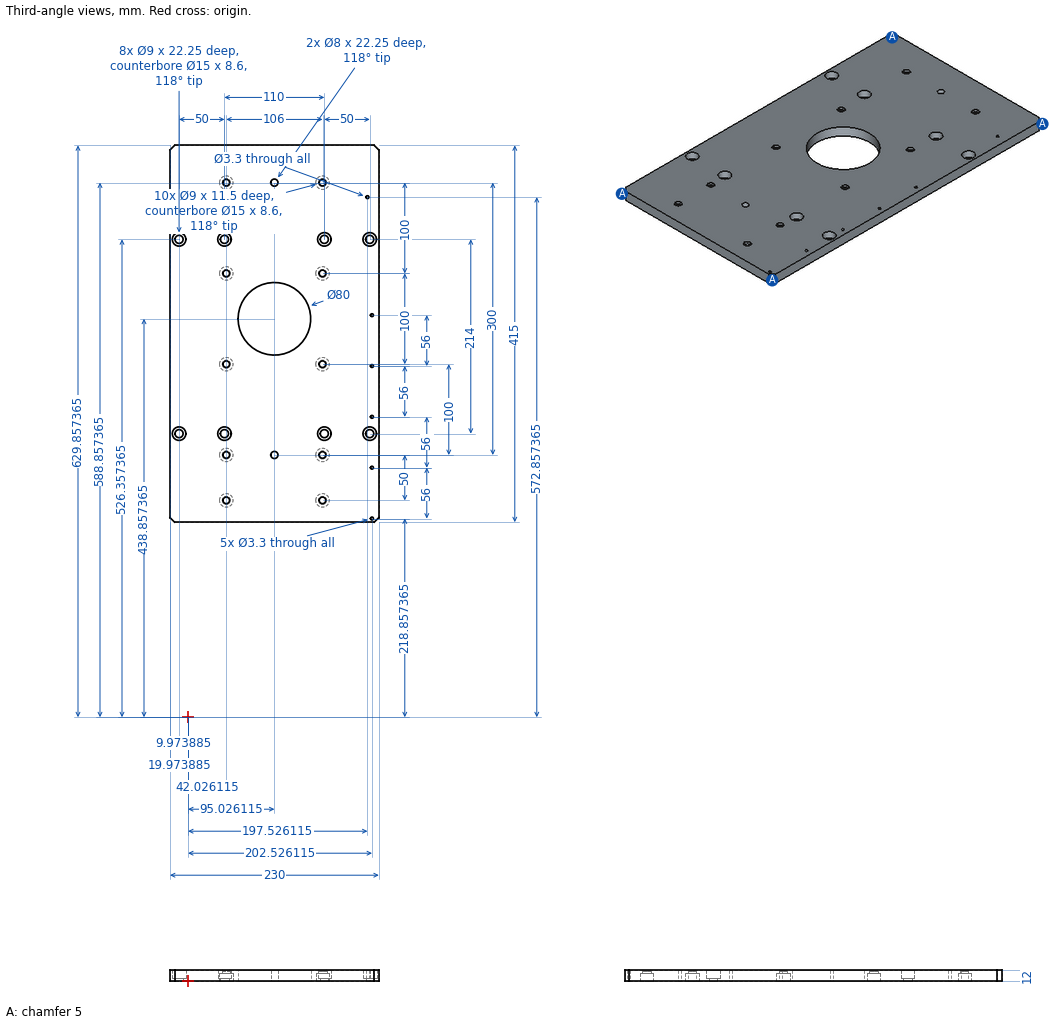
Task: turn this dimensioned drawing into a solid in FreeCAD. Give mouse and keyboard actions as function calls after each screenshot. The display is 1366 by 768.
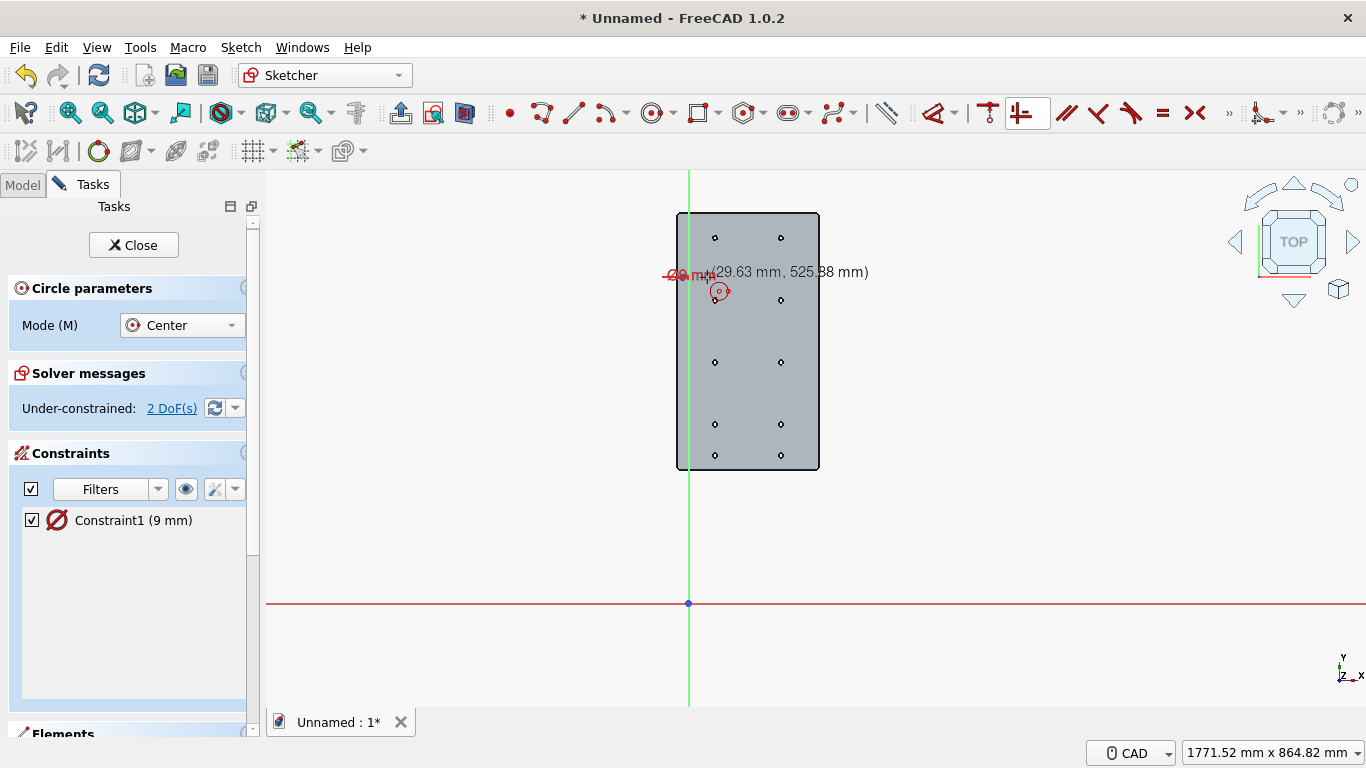
click(714, 277)
move(716, 275)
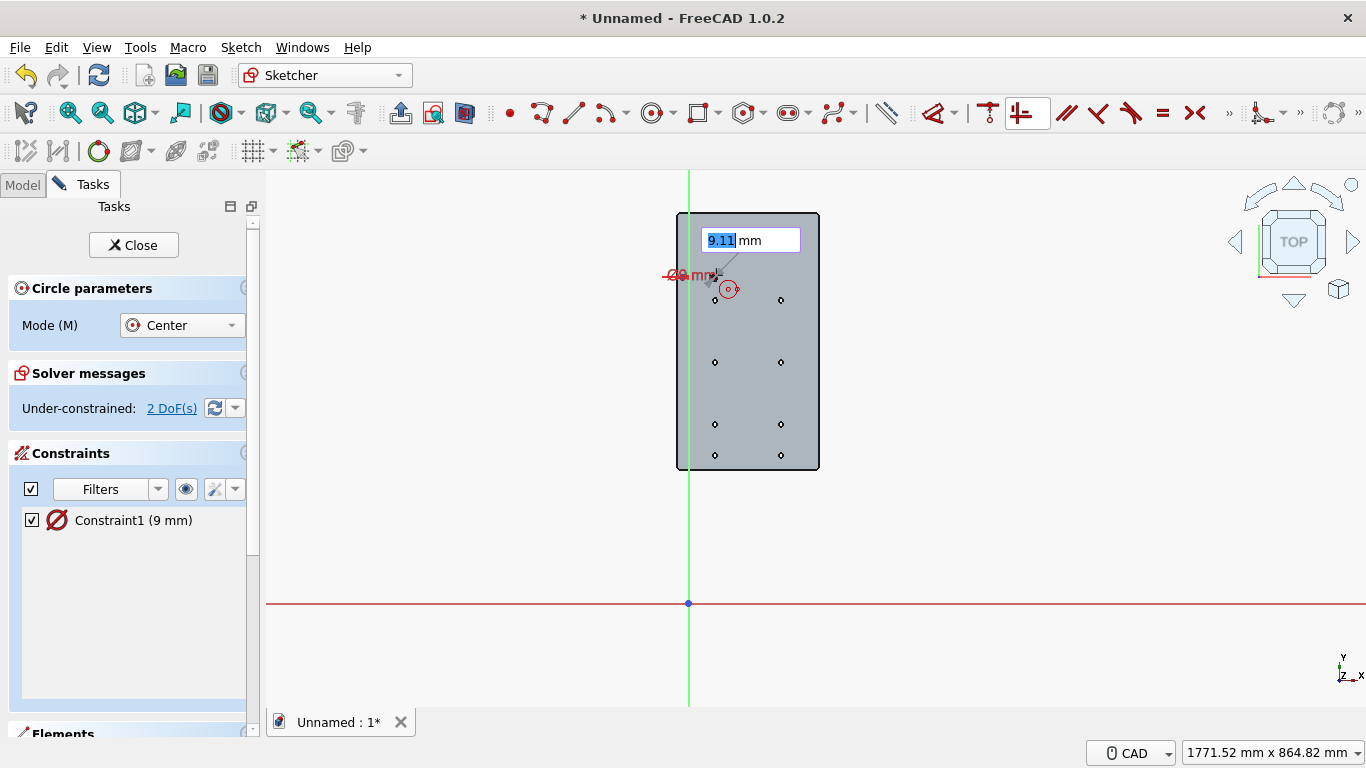
text(9)
key(Return)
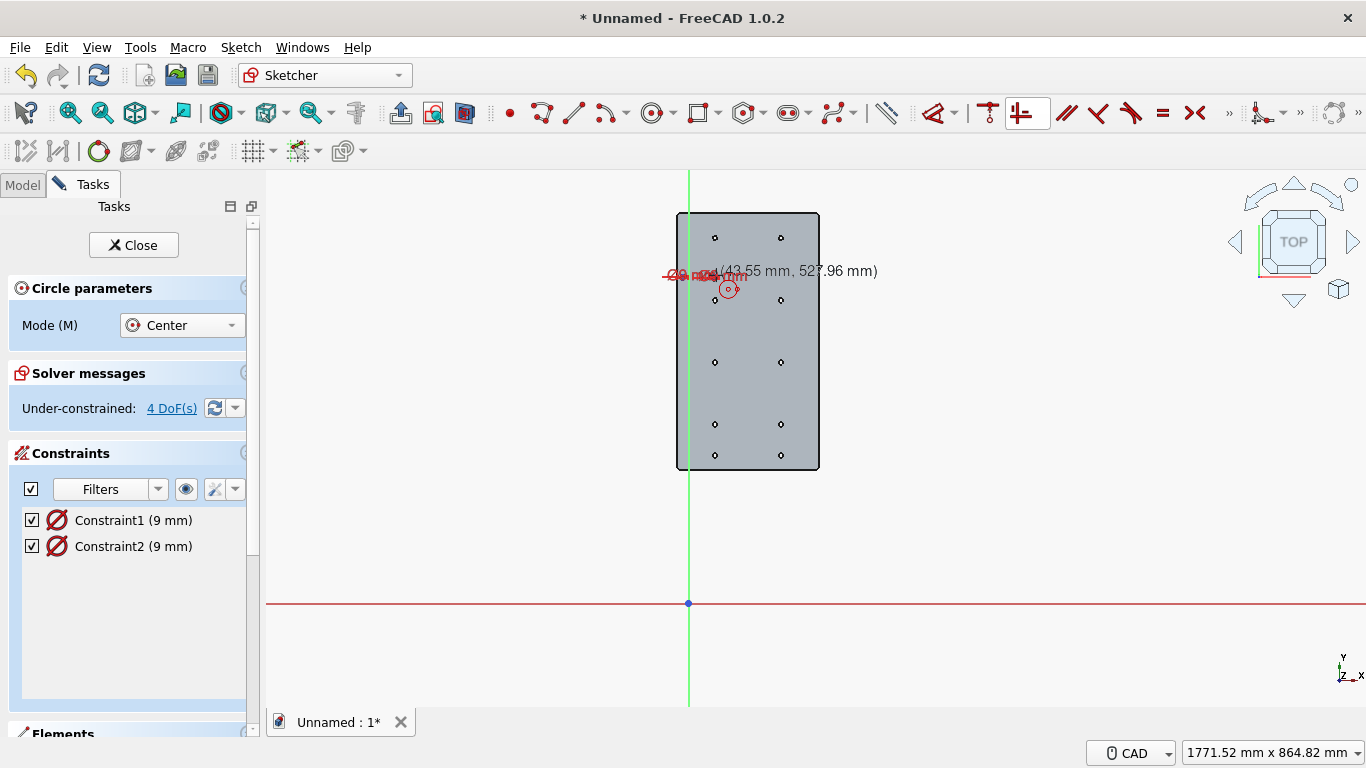
scroll(782, 277, up, 11)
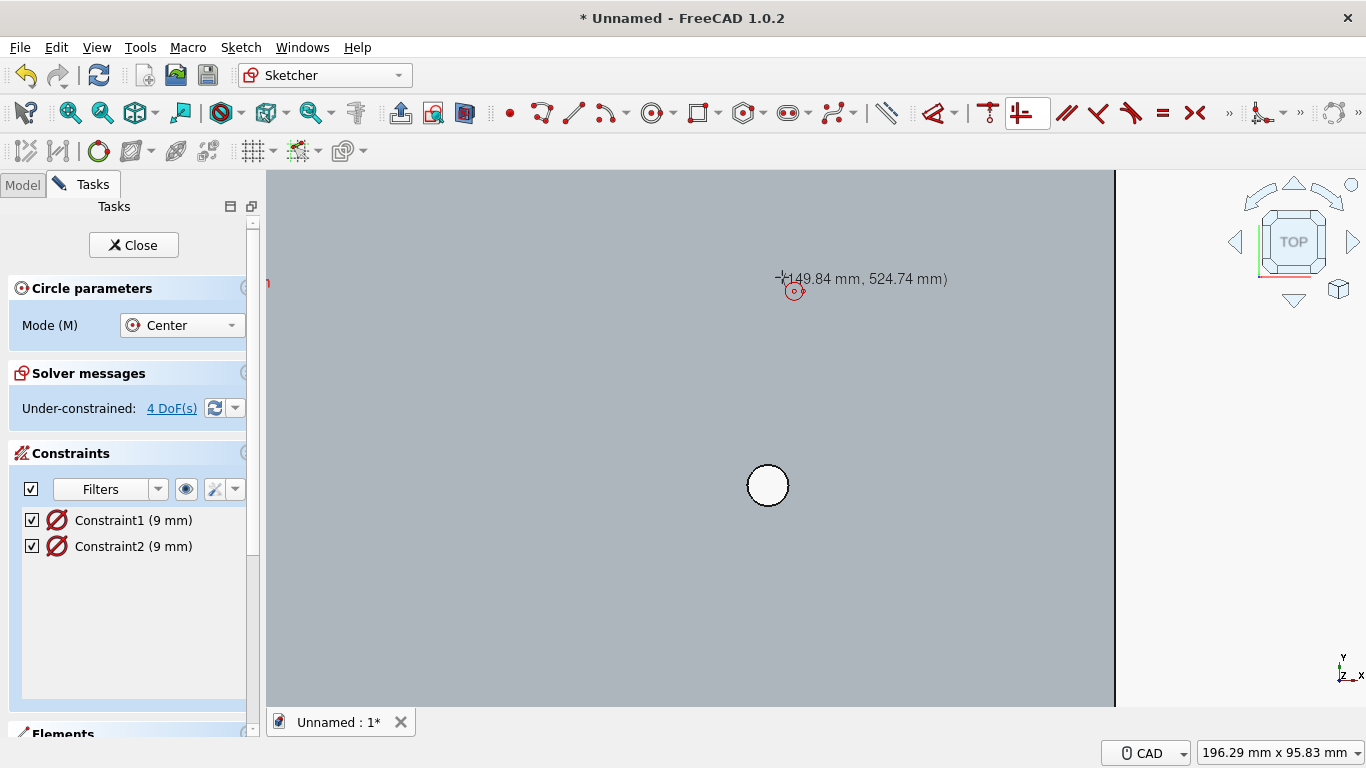
scroll(782, 277, down, 11)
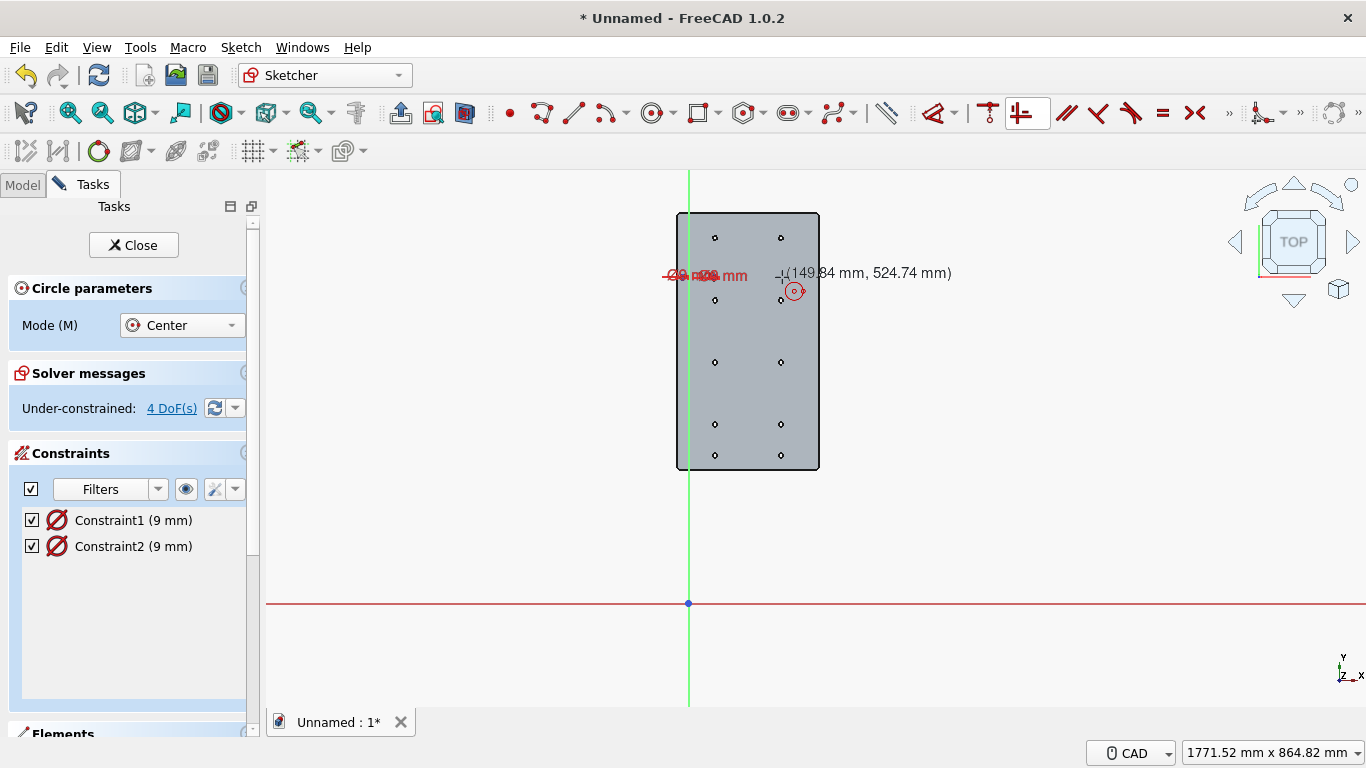
click(782, 277)
move(784, 275)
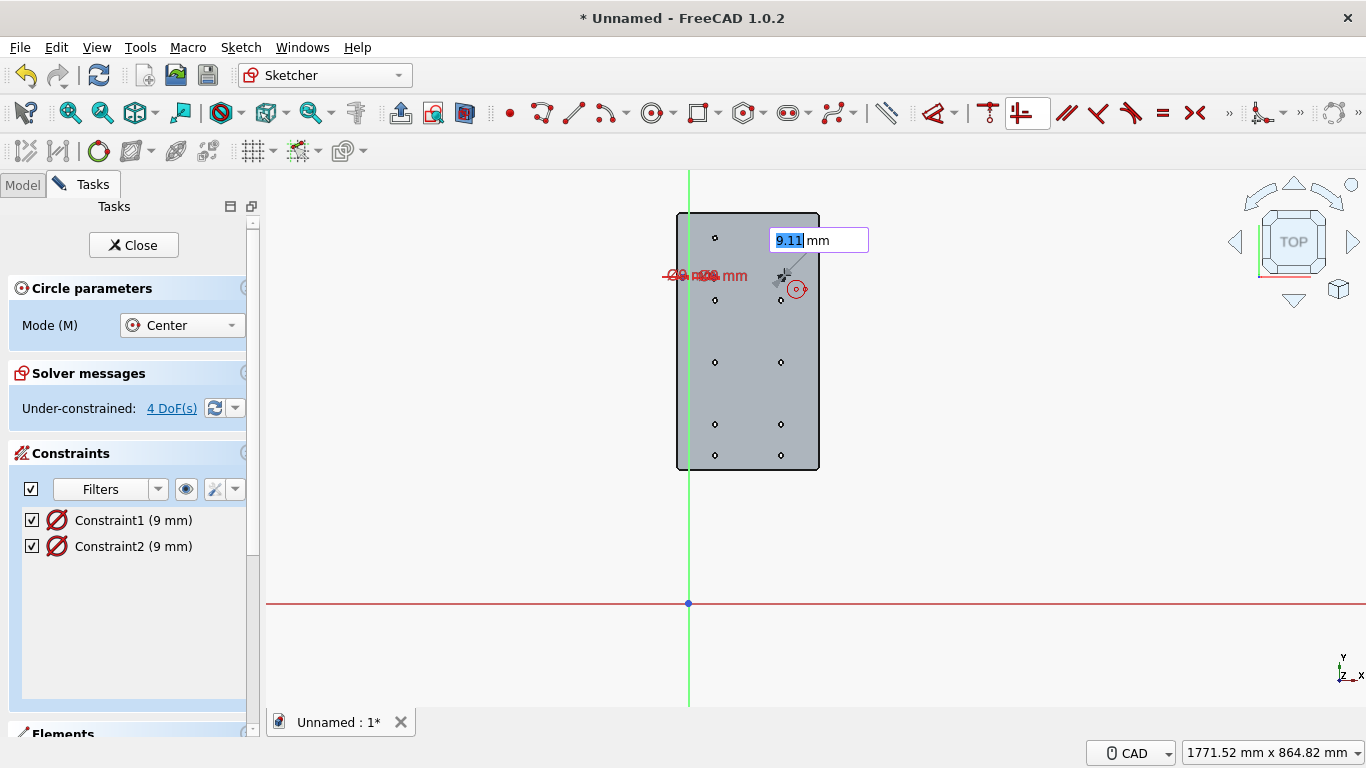
text(9)
key(Return)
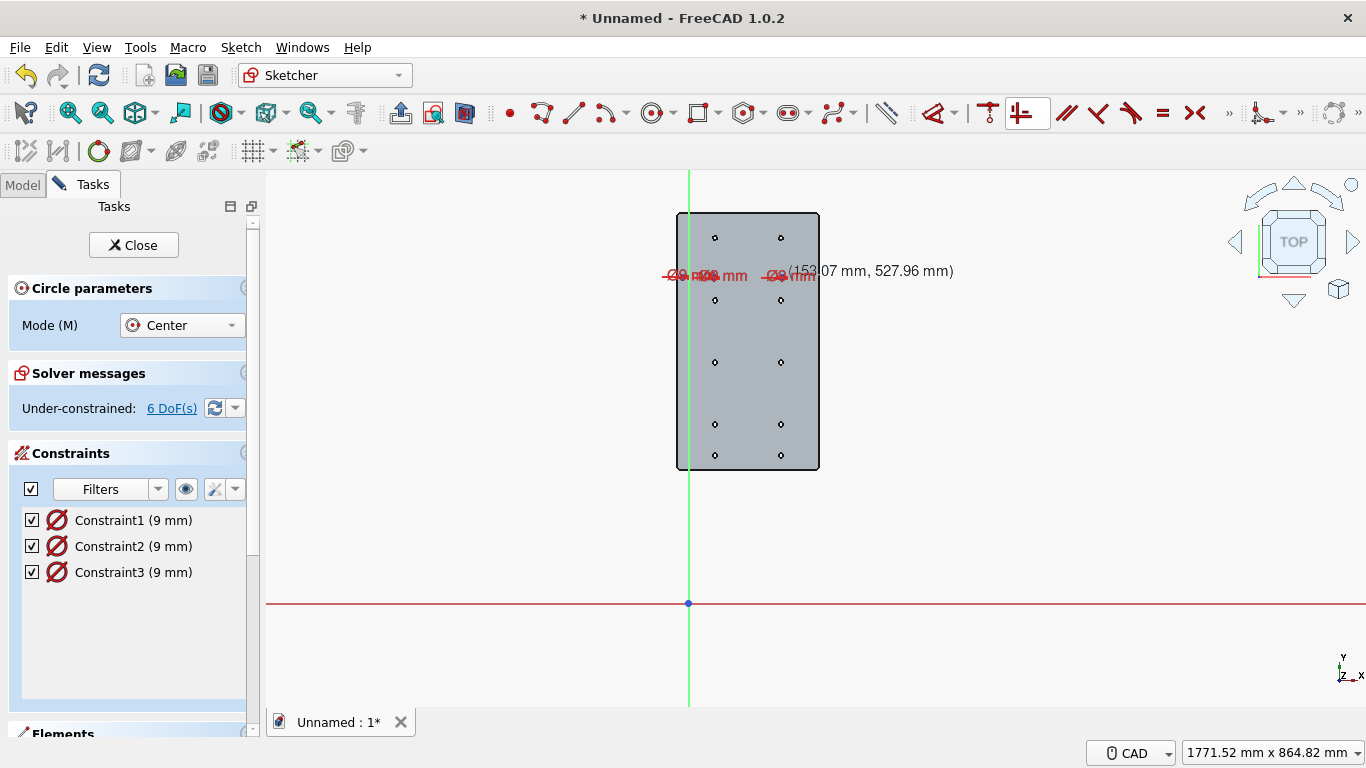
scroll(813, 277, up, 11)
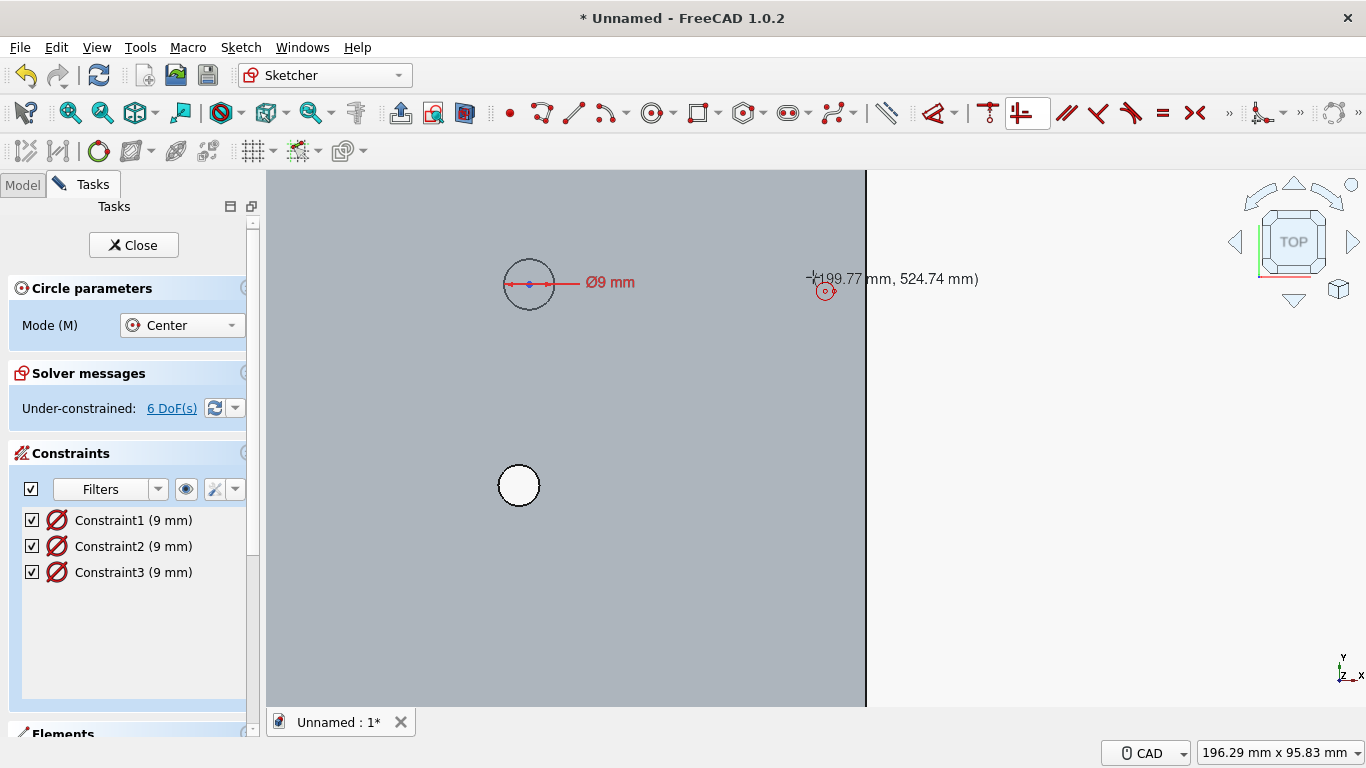
scroll(813, 277, down, 11)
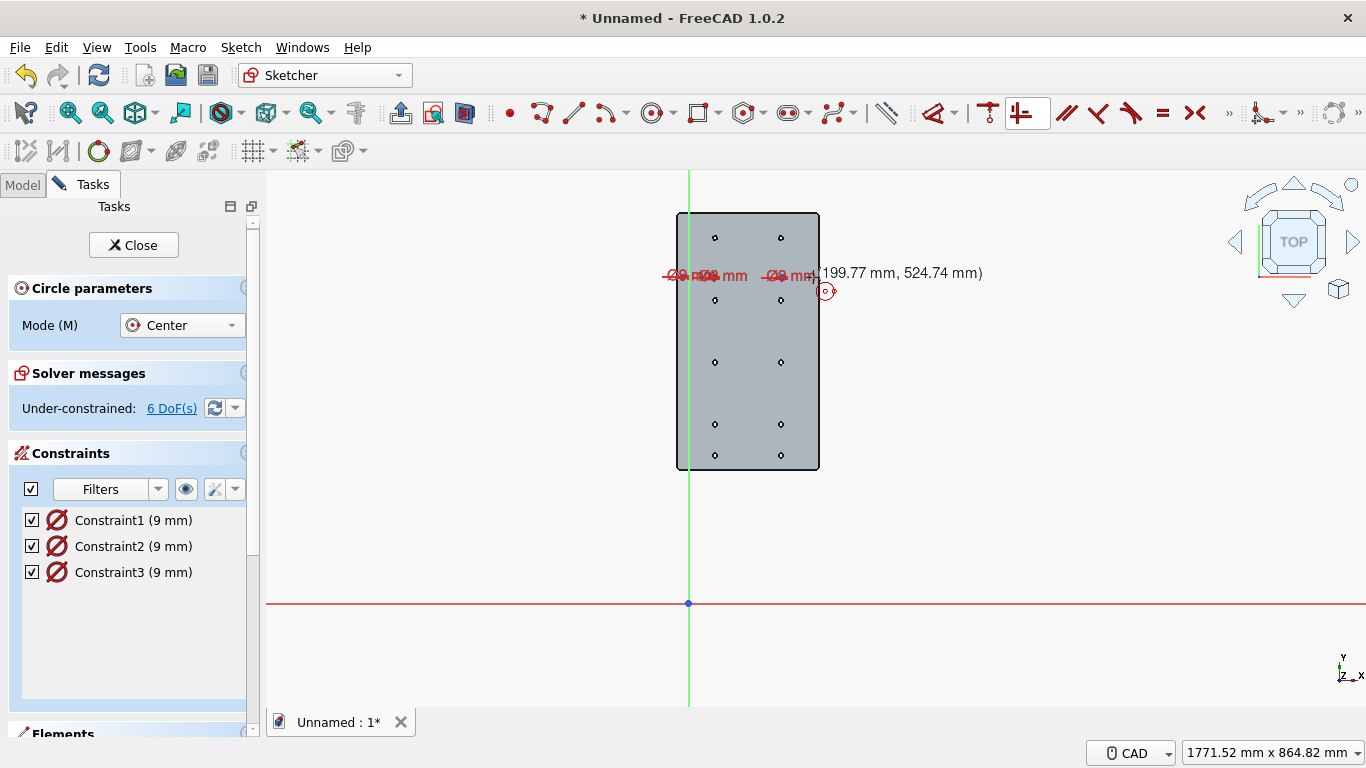
click(813, 277)
move(815, 275)